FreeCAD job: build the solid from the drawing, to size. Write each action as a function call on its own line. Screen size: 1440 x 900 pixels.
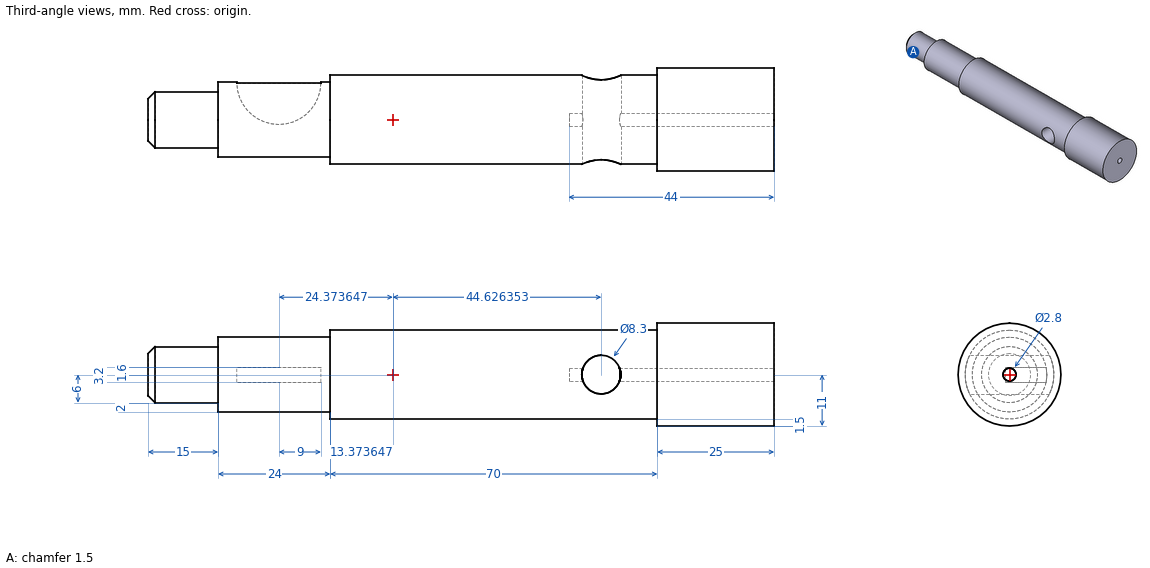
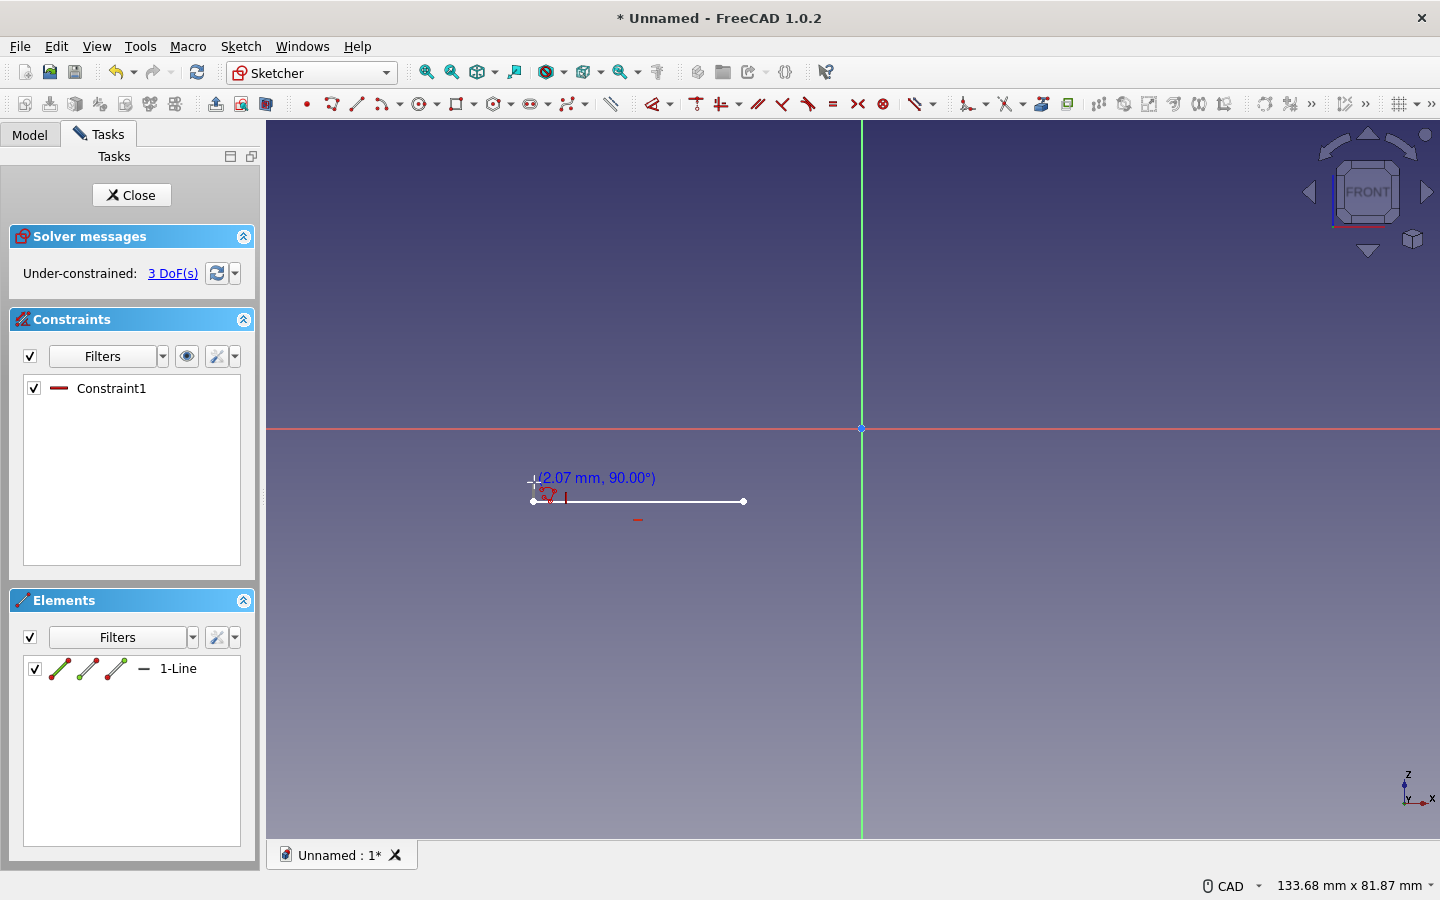
click(534, 482)
click(402, 482)
click(402, 429)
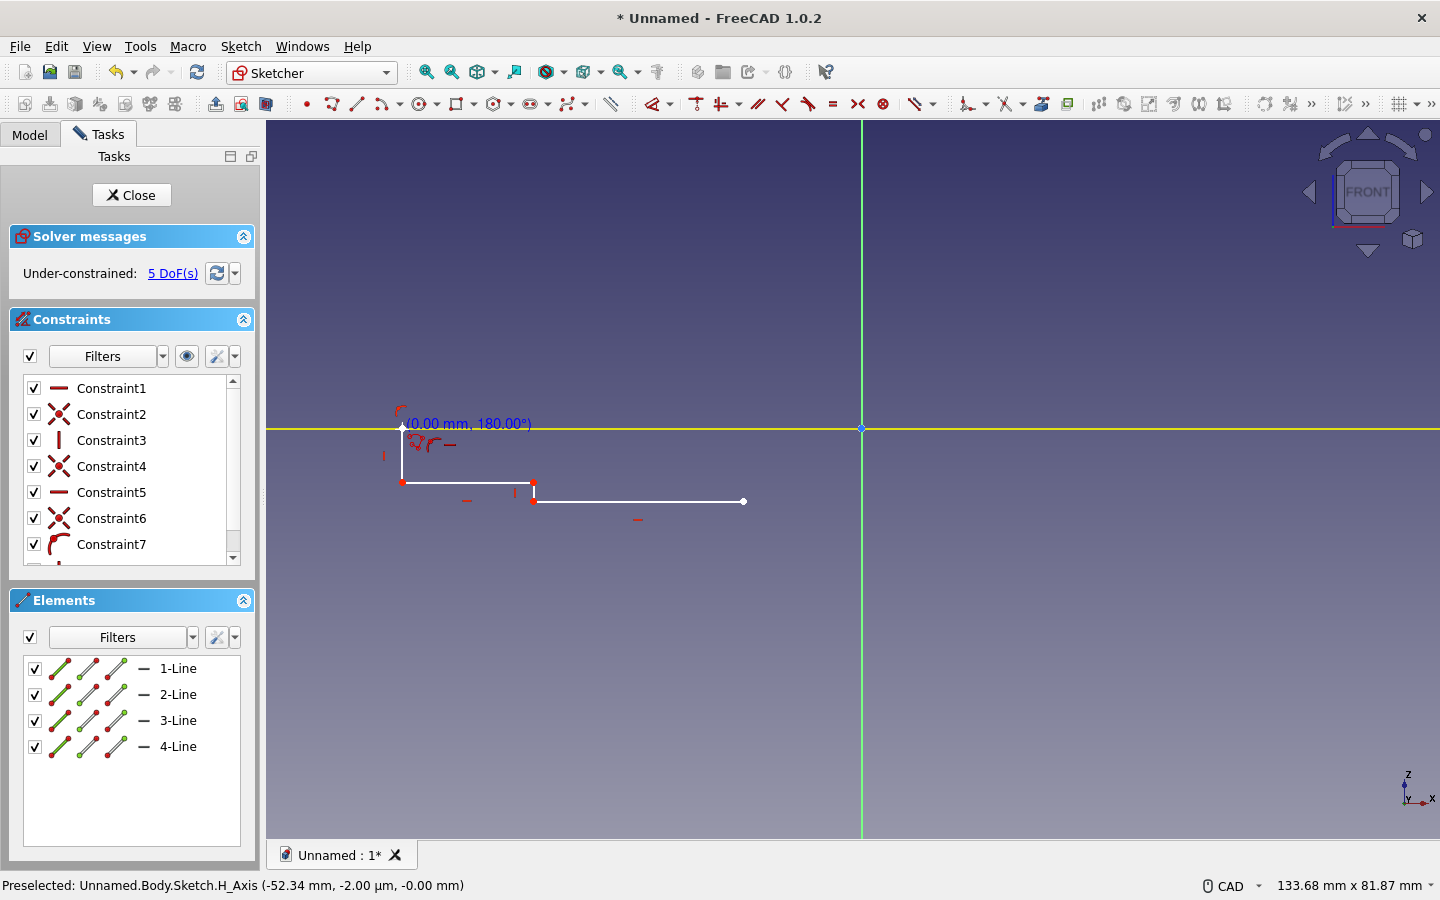
scroll(534, 482, down, 3)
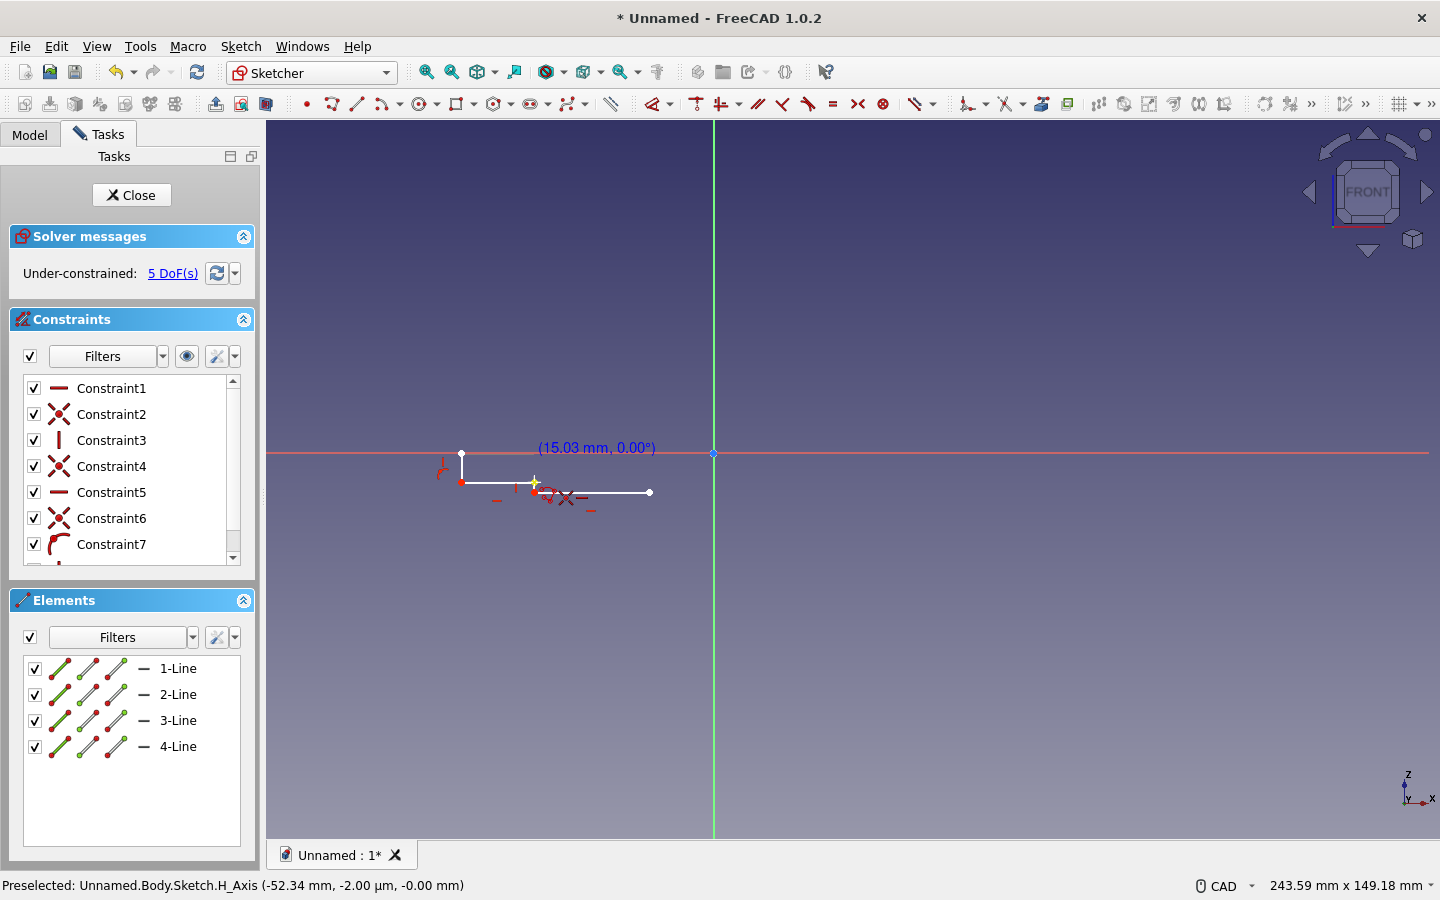
click(1107, 462)
click(1107, 506)
click(987, 506)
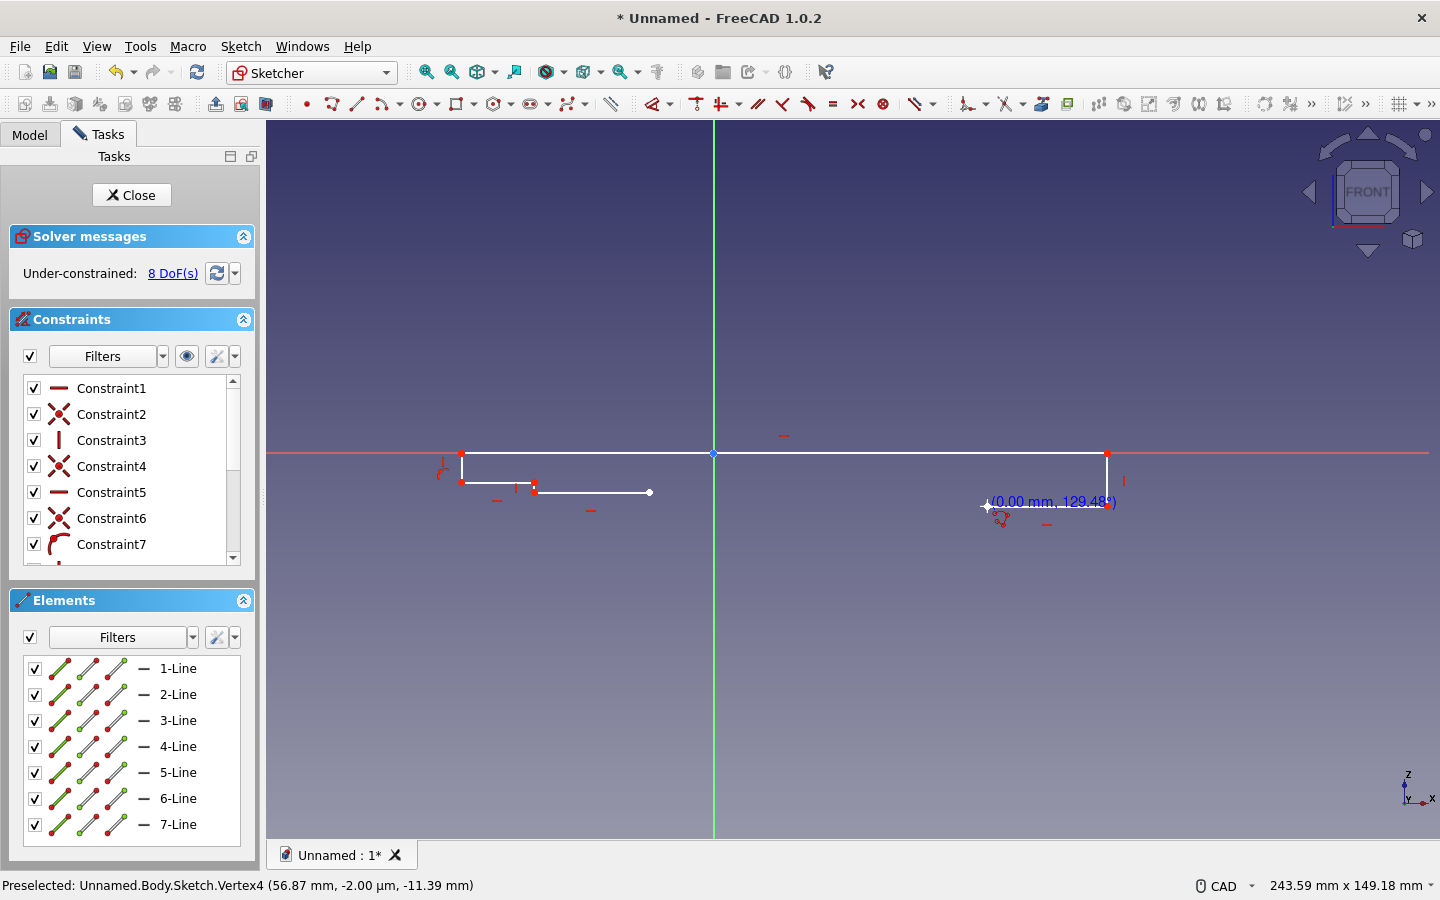
scroll(987, 499, up, 4)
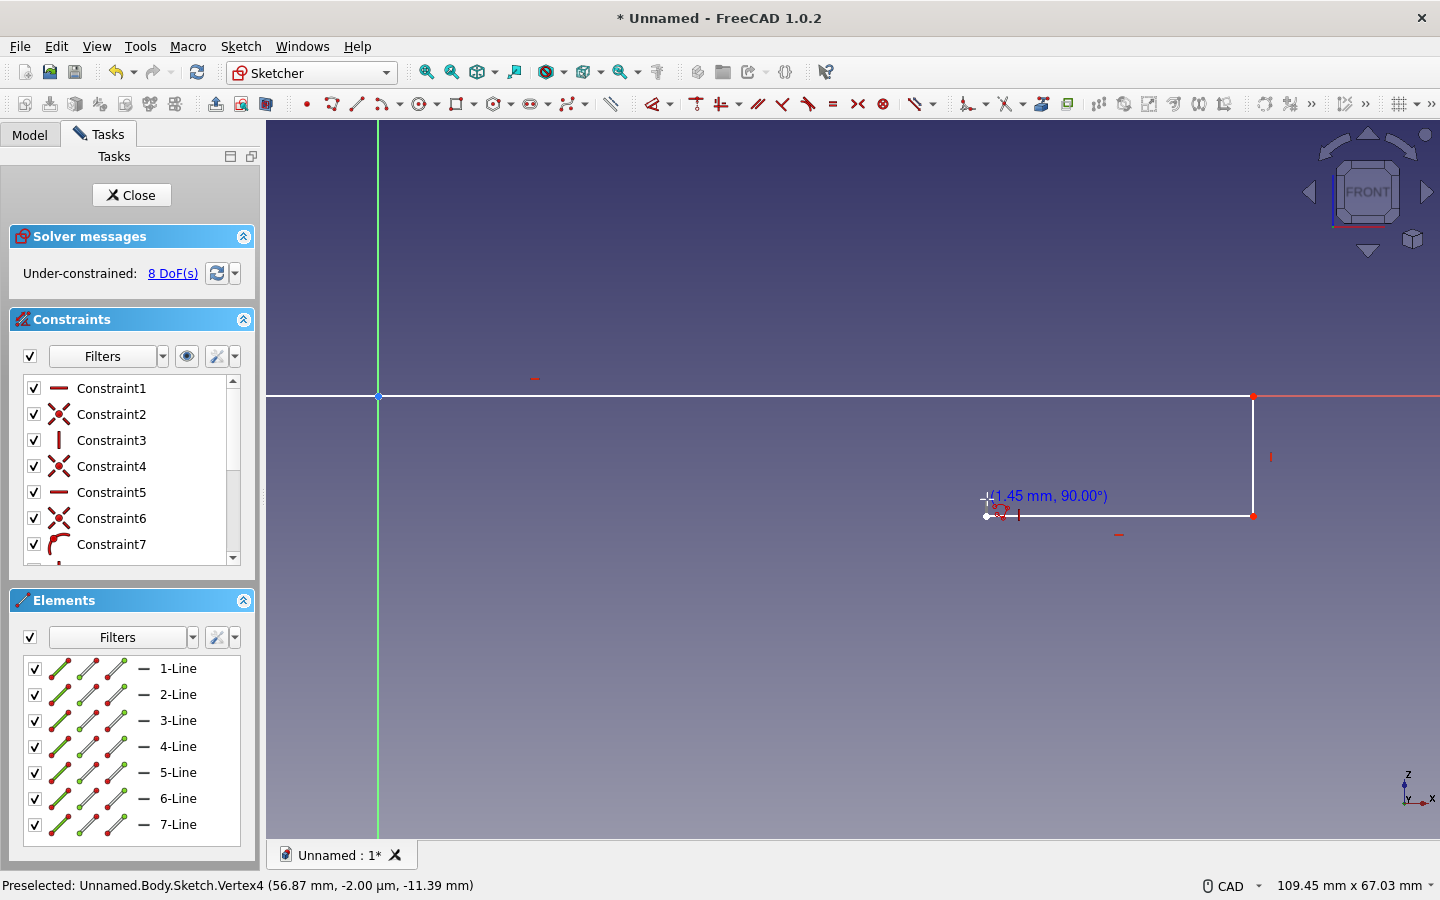
click(986, 498)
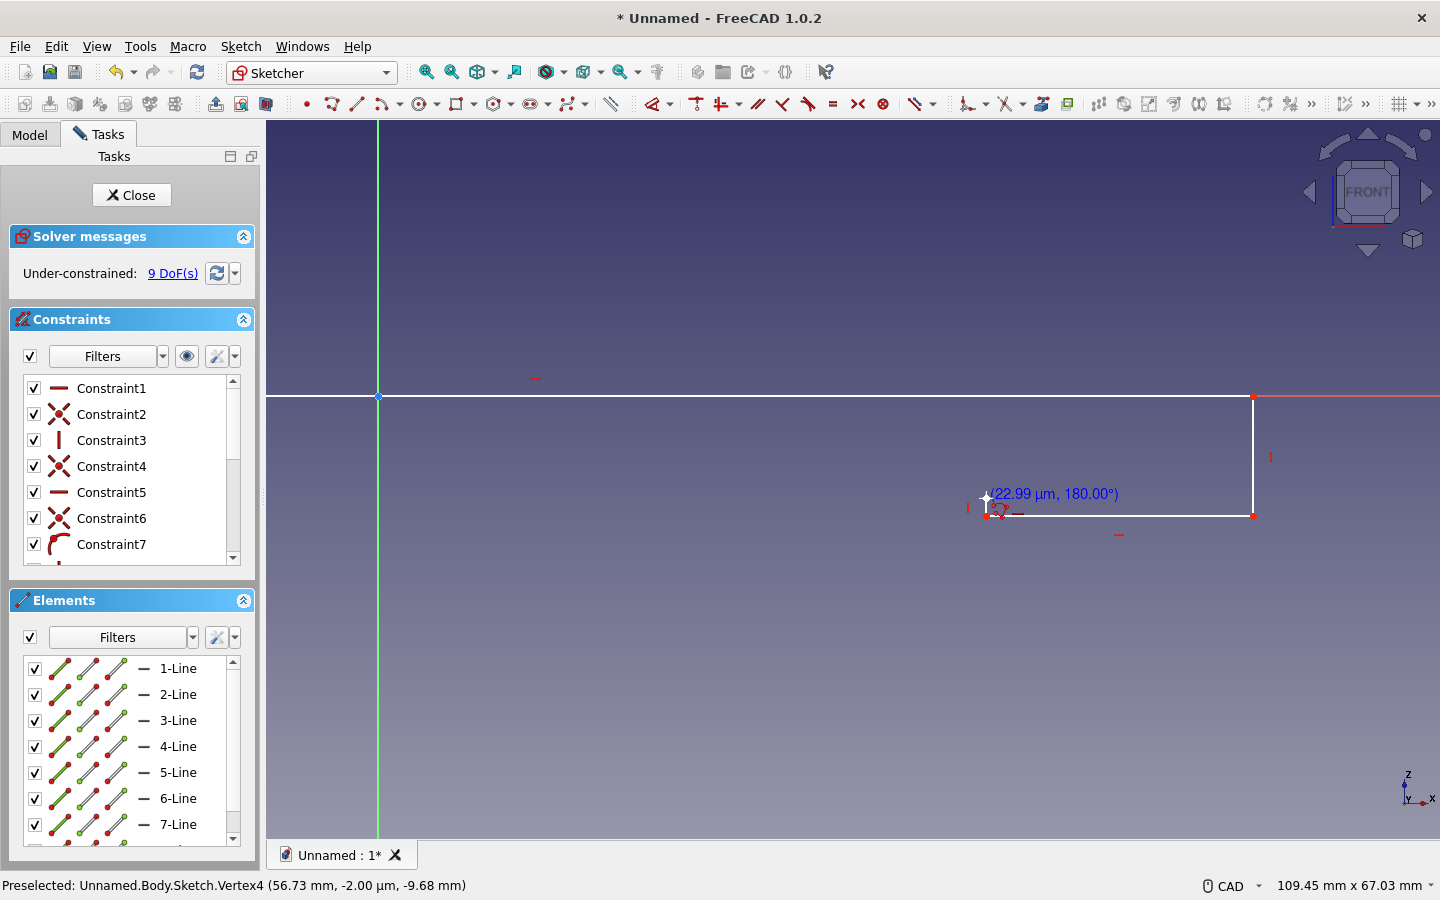
scroll(988, 499, down, 4)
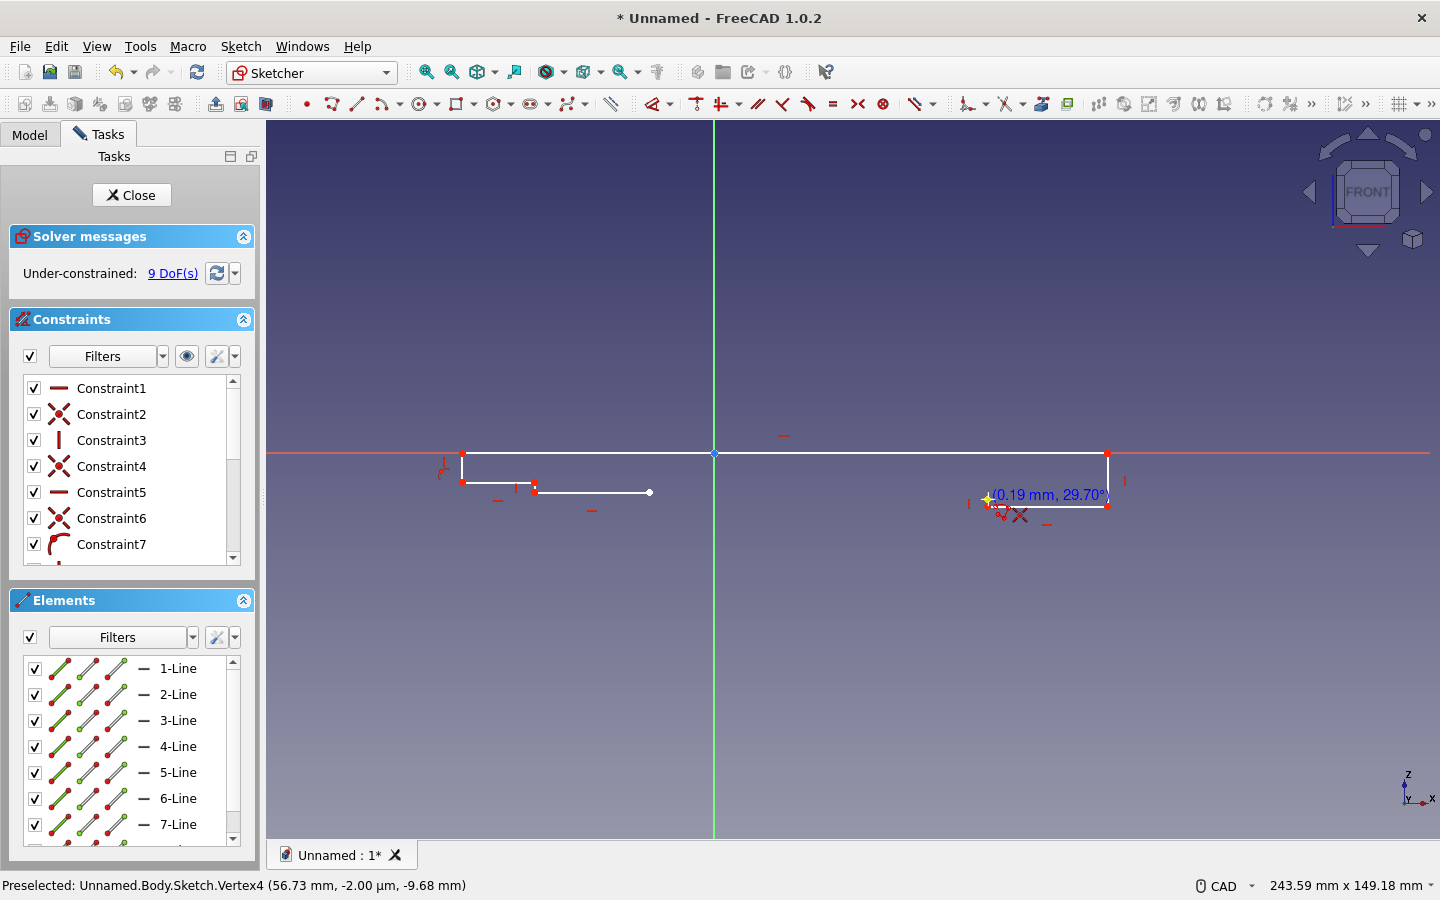
scroll(650, 499, up, 4)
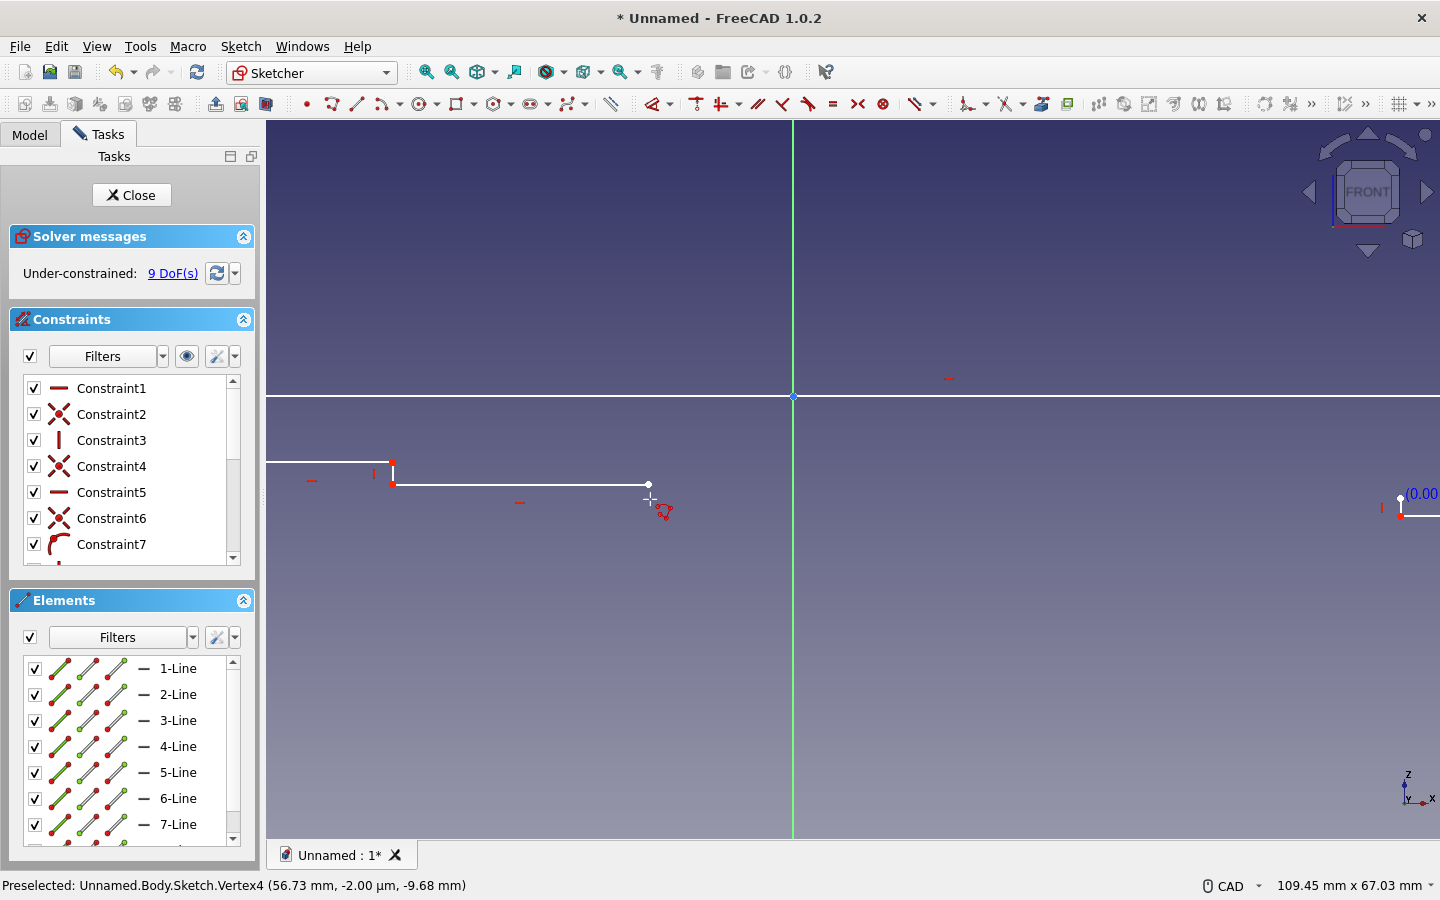
click(650, 498)
click(649, 485)
key(Escape)
key(Escape)